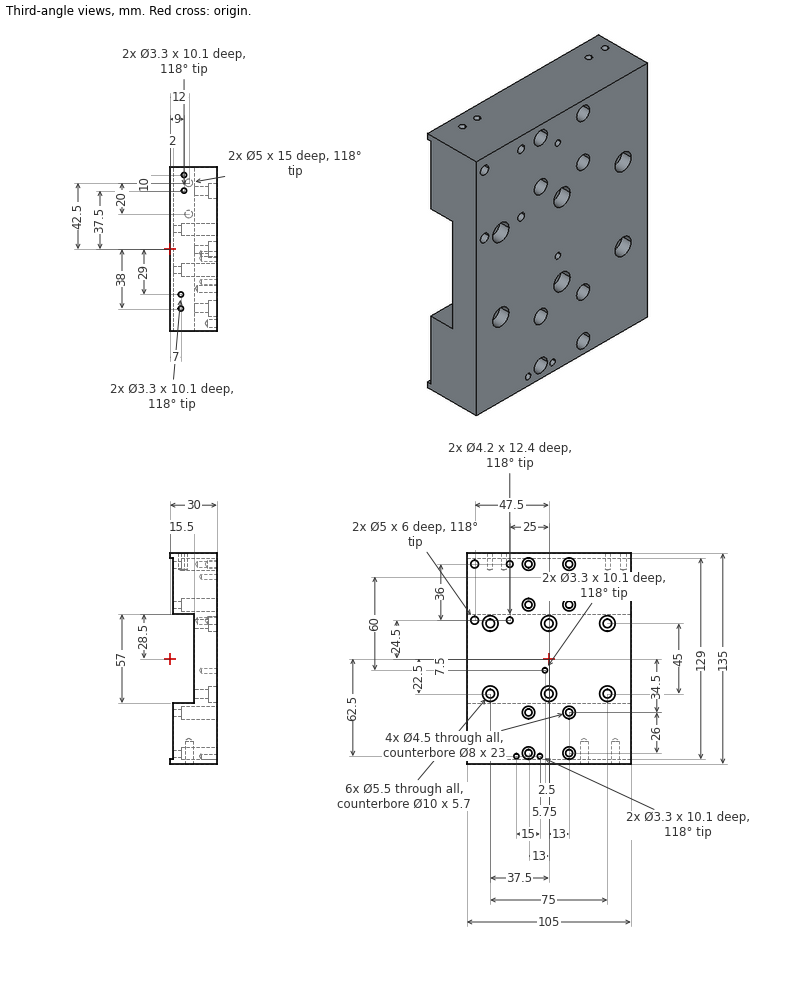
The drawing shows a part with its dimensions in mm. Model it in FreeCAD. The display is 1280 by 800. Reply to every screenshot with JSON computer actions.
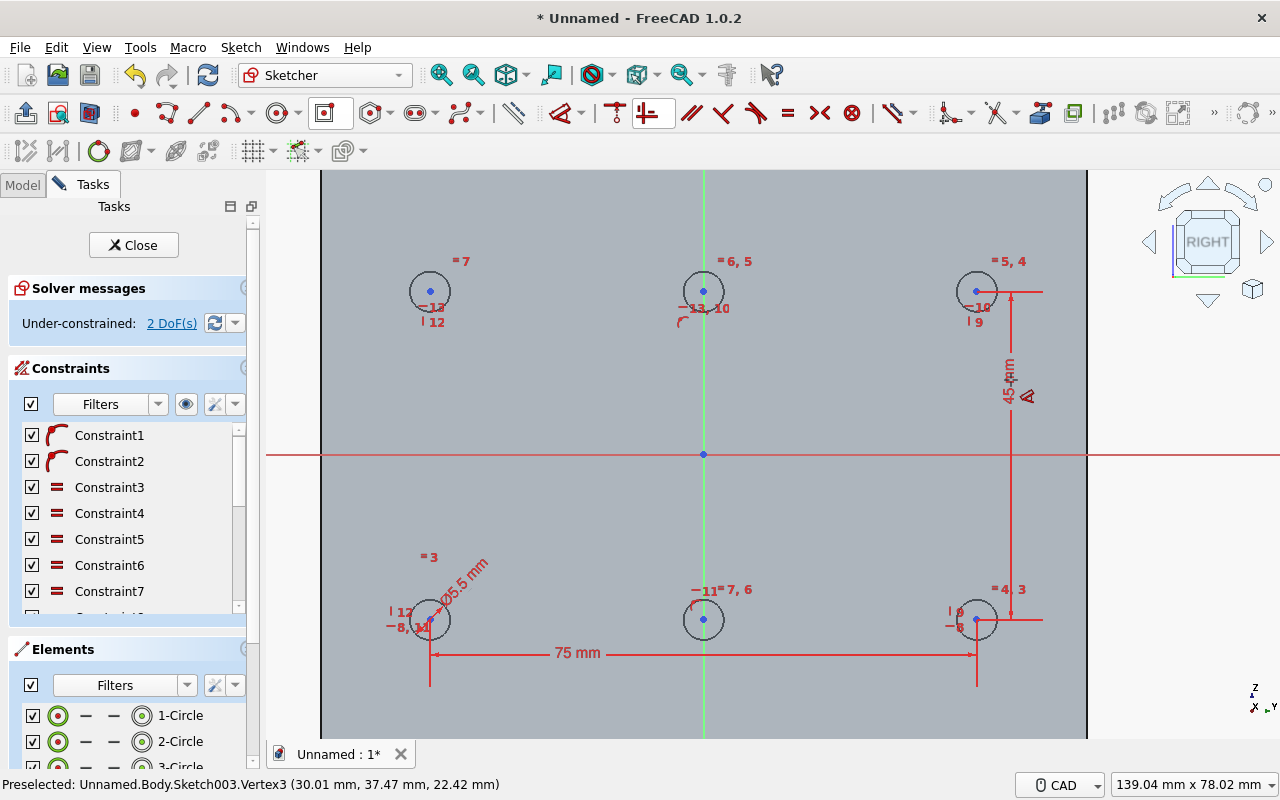
{"action": "left_click", "coordinate": [430, 620]}
{"action": "left_click", "coordinate": [504, 654]}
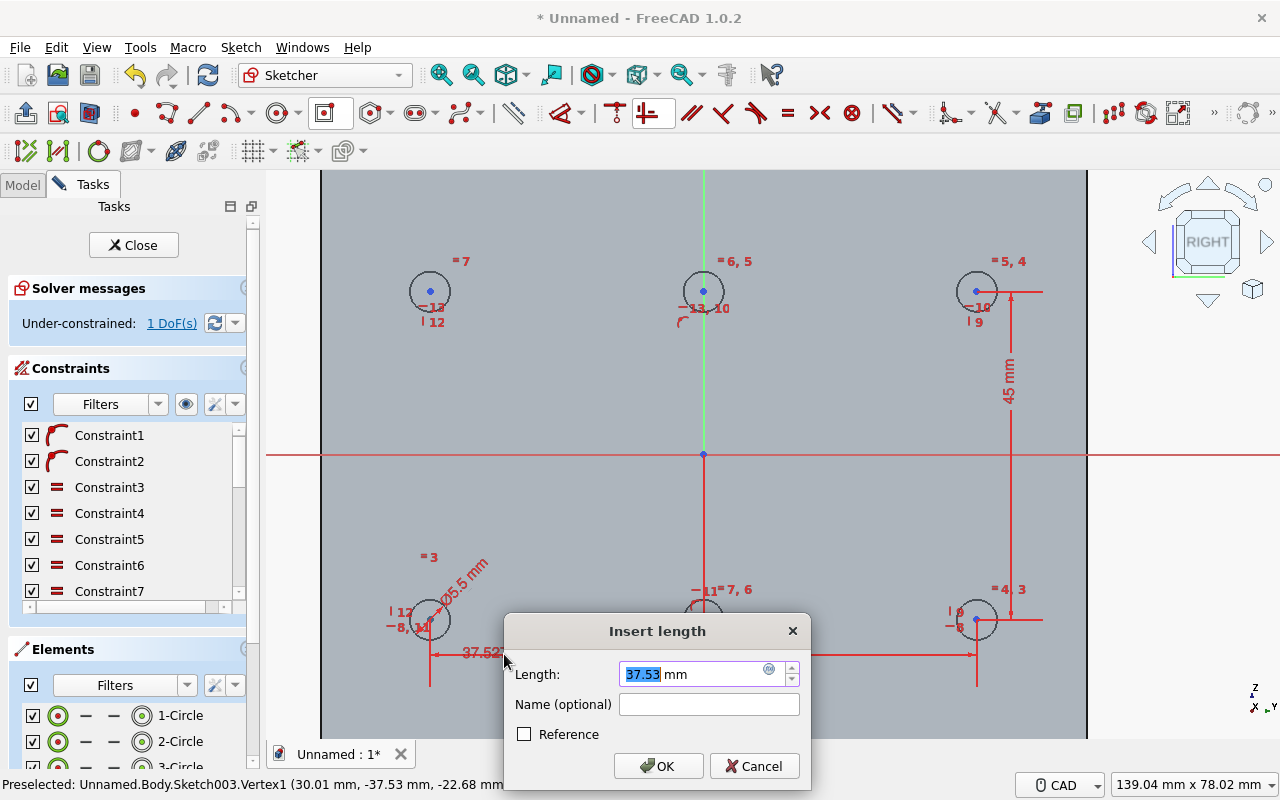
{"action": "type", "text": "37.5"}
{"action": "key", "text": "Return"}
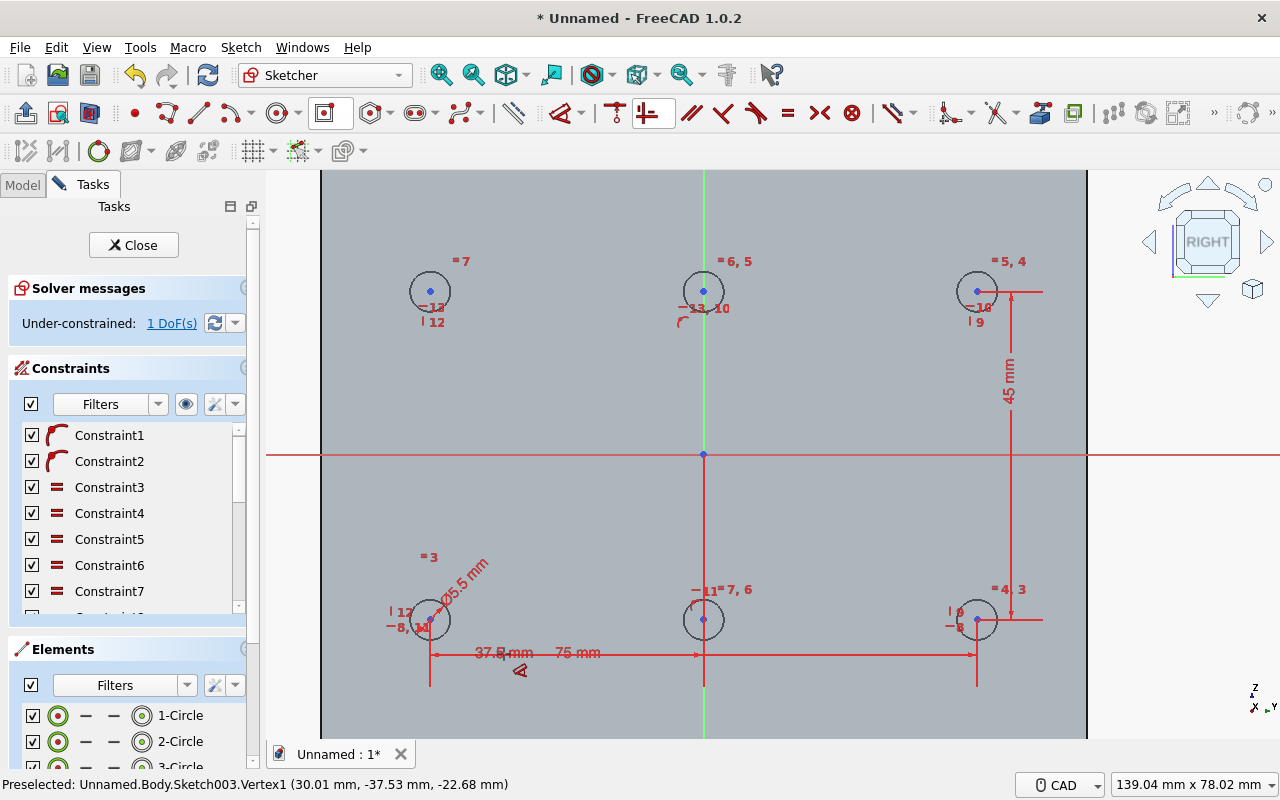
{"action": "left_click", "coordinate": [430, 620]}
{"action": "left_click", "coordinate": [396, 537]}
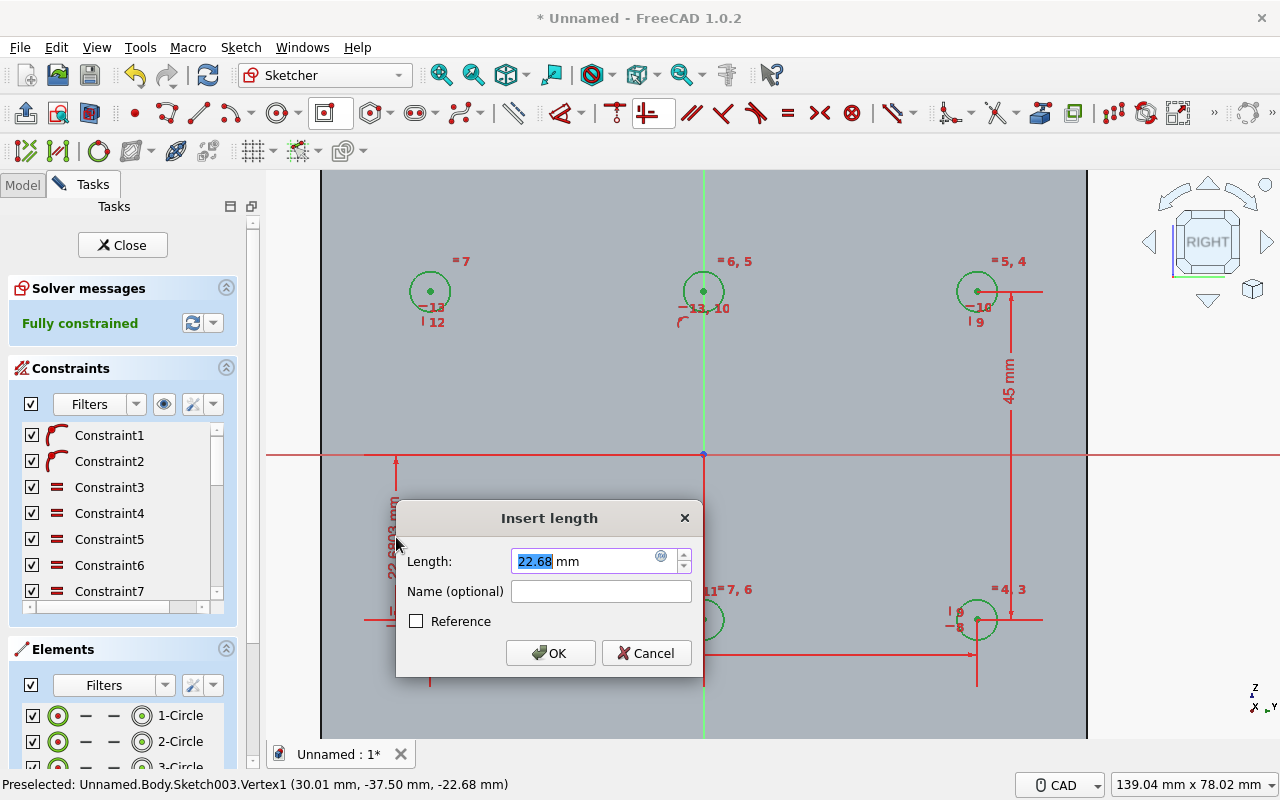
{"action": "type", "text": "22.5"}
{"action": "key", "text": "Return"}
{"action": "key", "text": "Escape"}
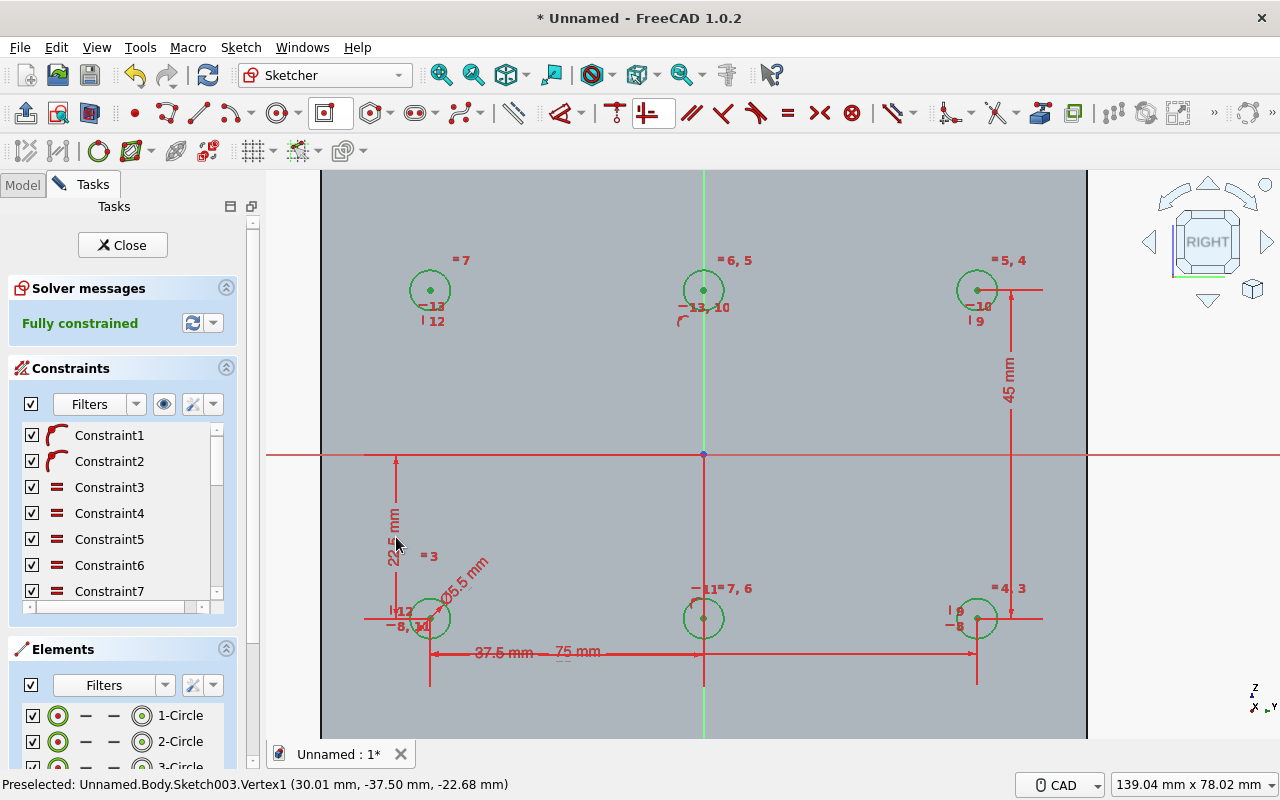
{"action": "left_click", "coordinate": [123, 245]}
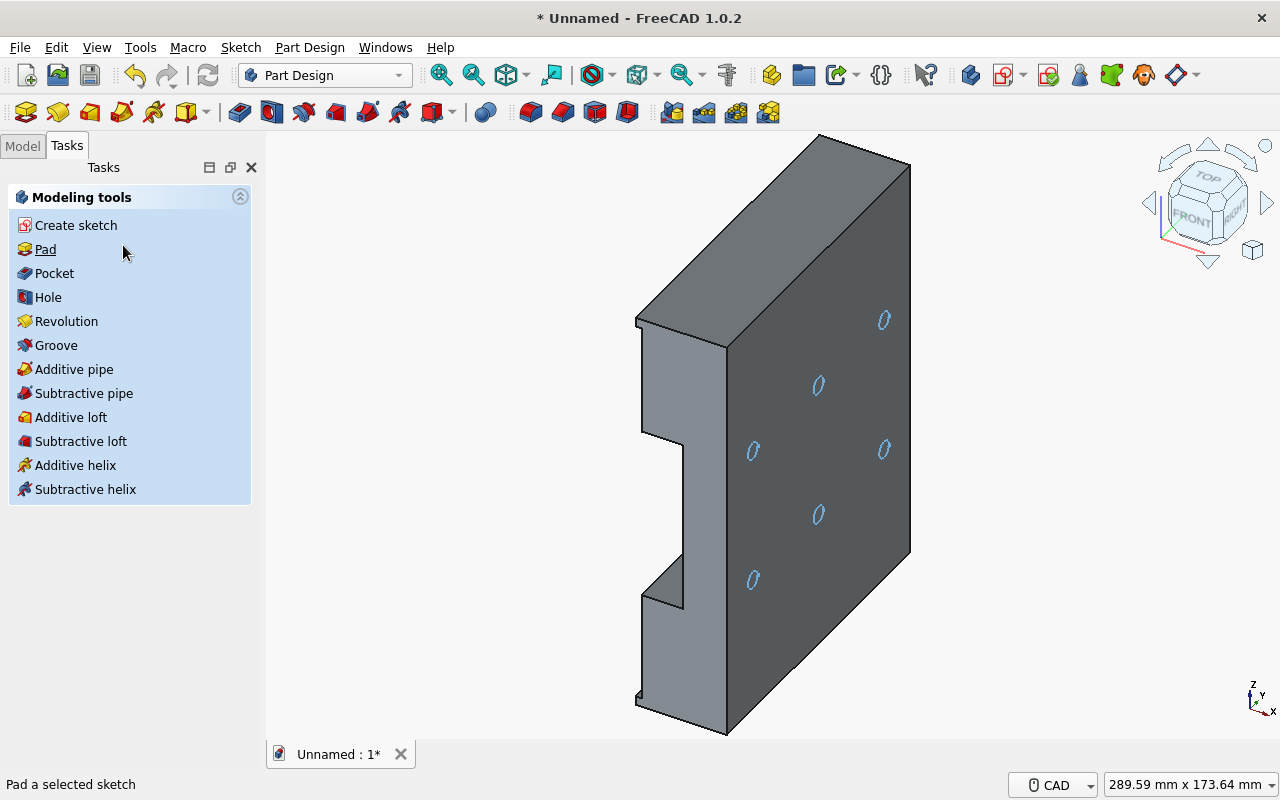
{"action": "left_click", "coordinate": [272, 112]}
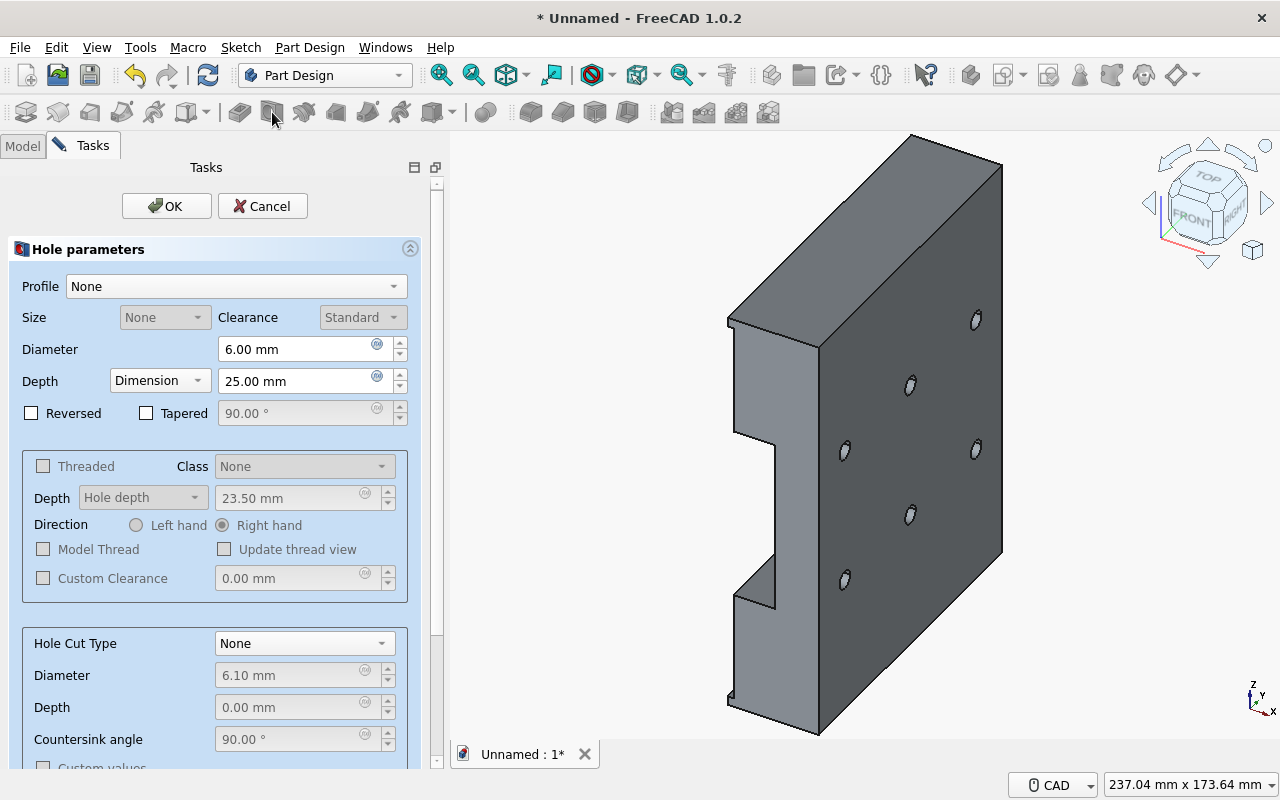
{"action": "triple_click", "coordinate": [305, 349]}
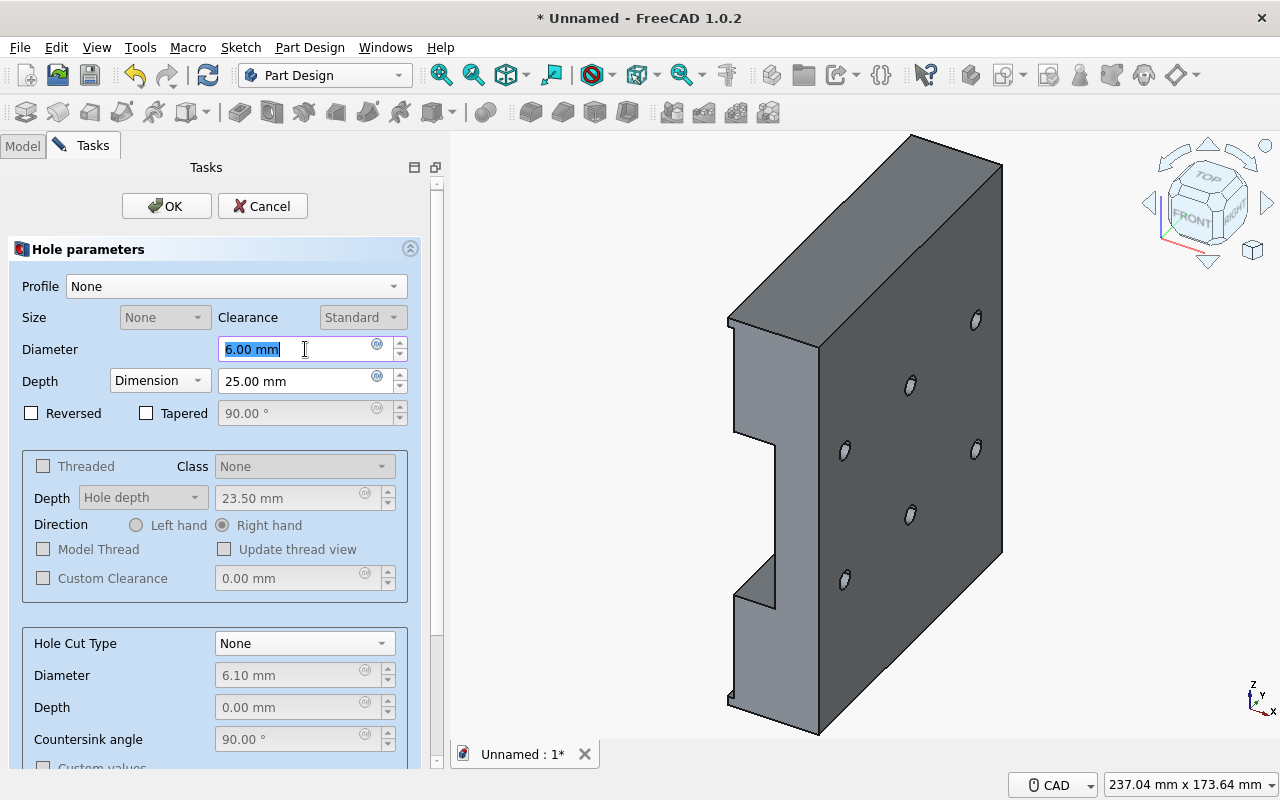
{"action": "type", "text": "5.5"}
{"action": "key", "text": "Tab"}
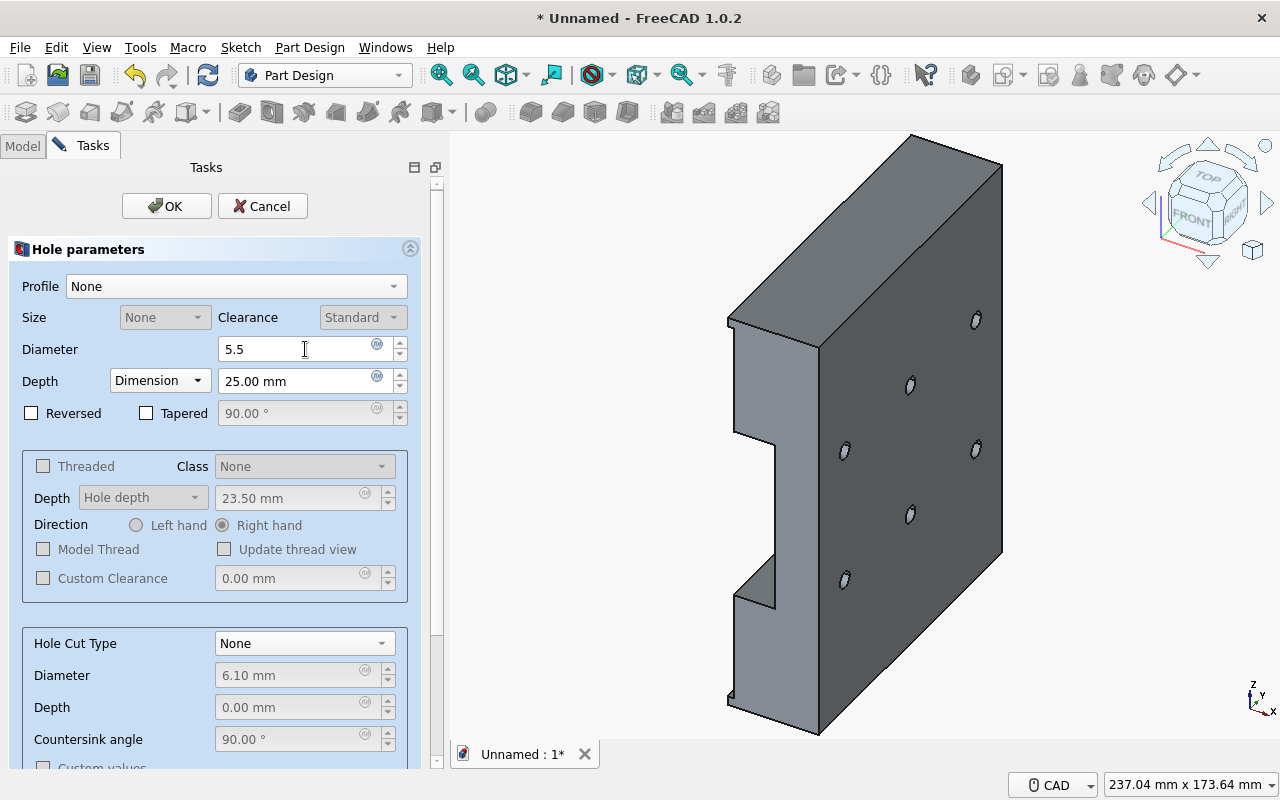
{"action": "left_click", "coordinate": [161, 380]}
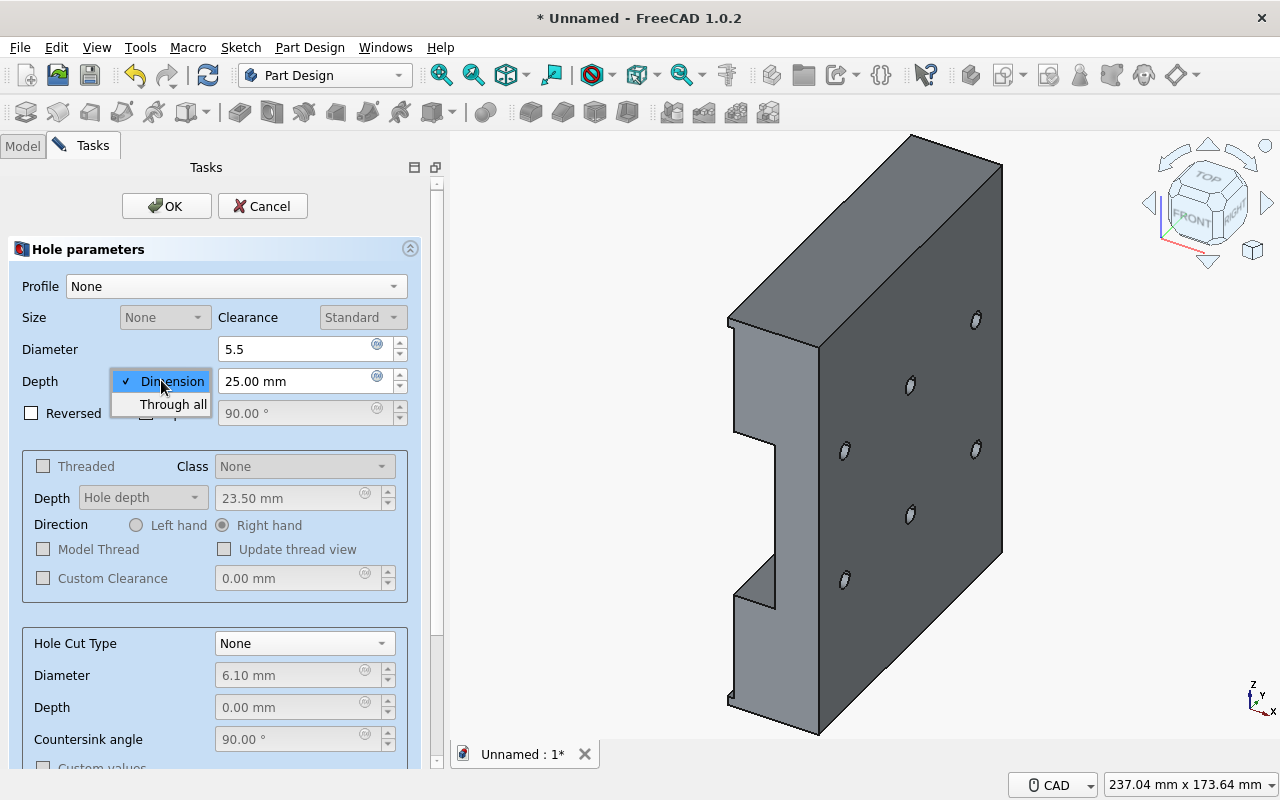
{"action": "left_click", "coordinate": [160, 404]}